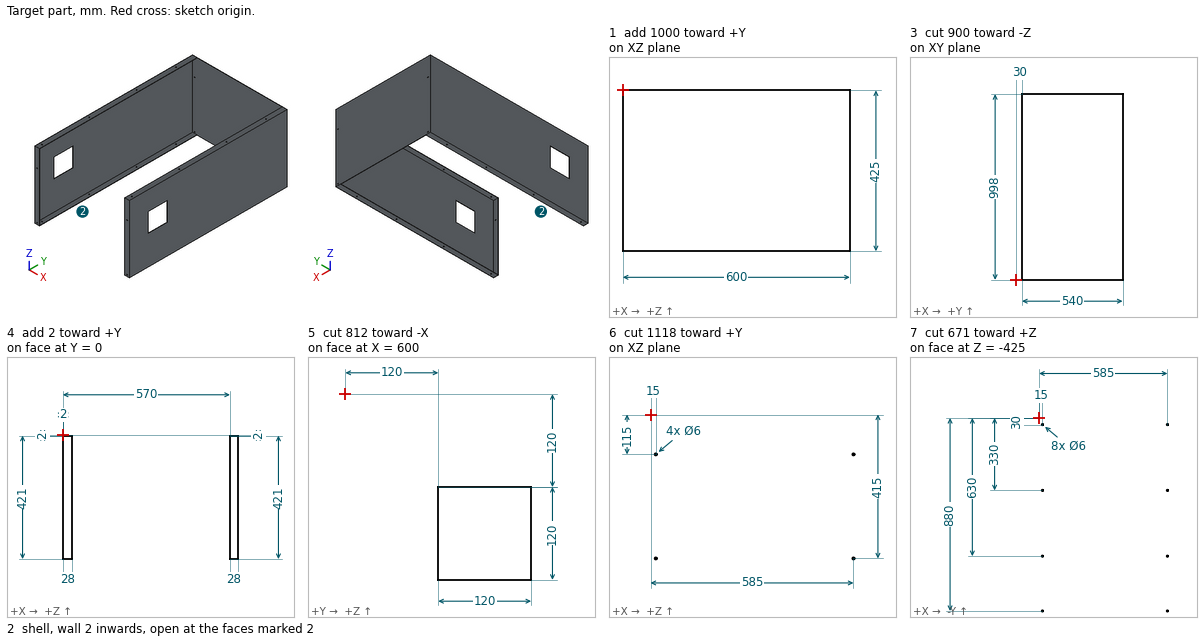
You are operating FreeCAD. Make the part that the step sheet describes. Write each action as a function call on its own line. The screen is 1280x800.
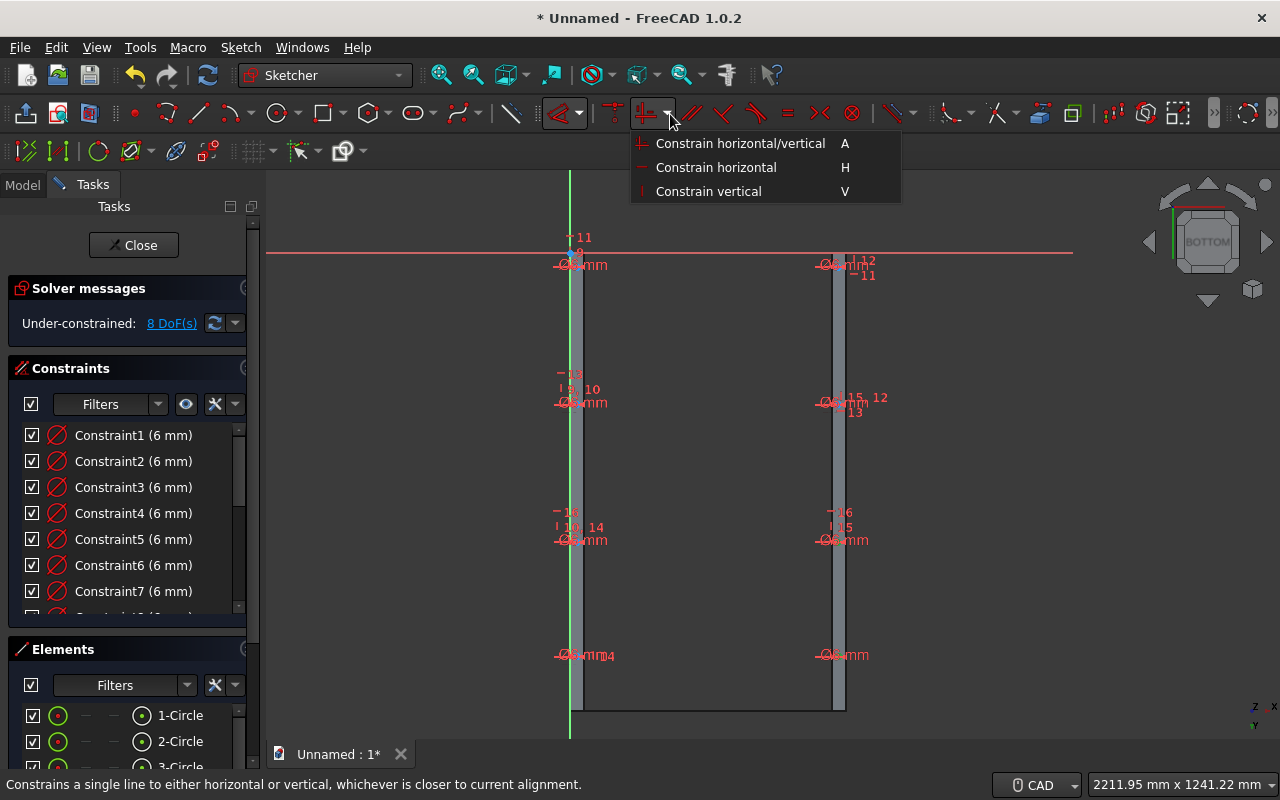
click(766, 191)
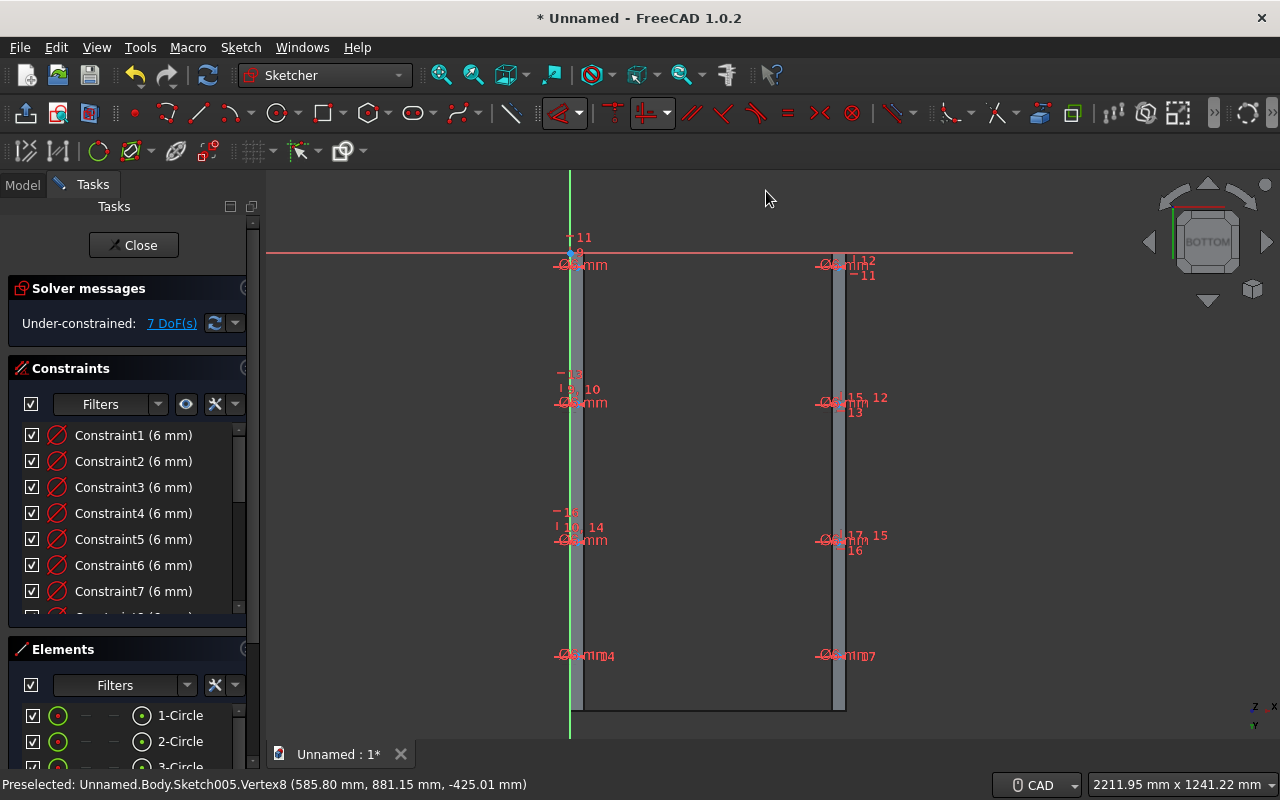
click(577, 657)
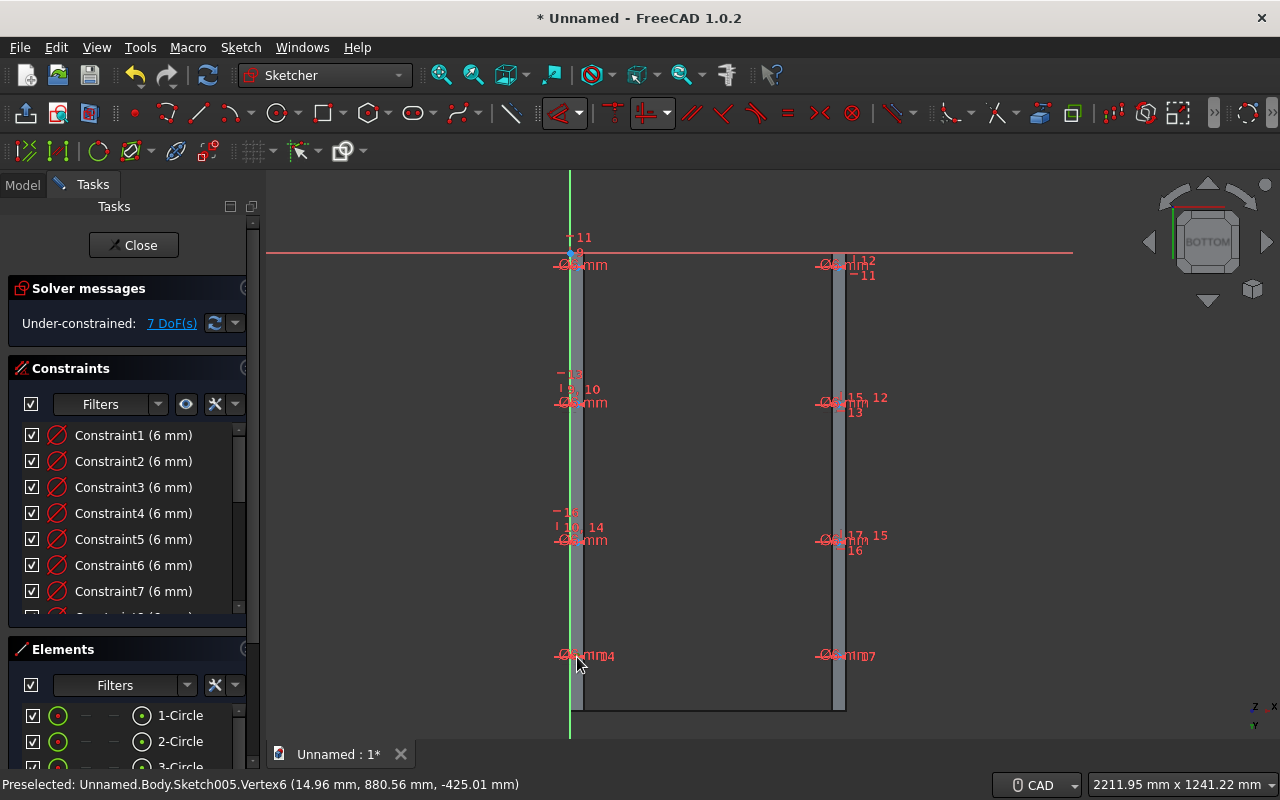
click(838, 657)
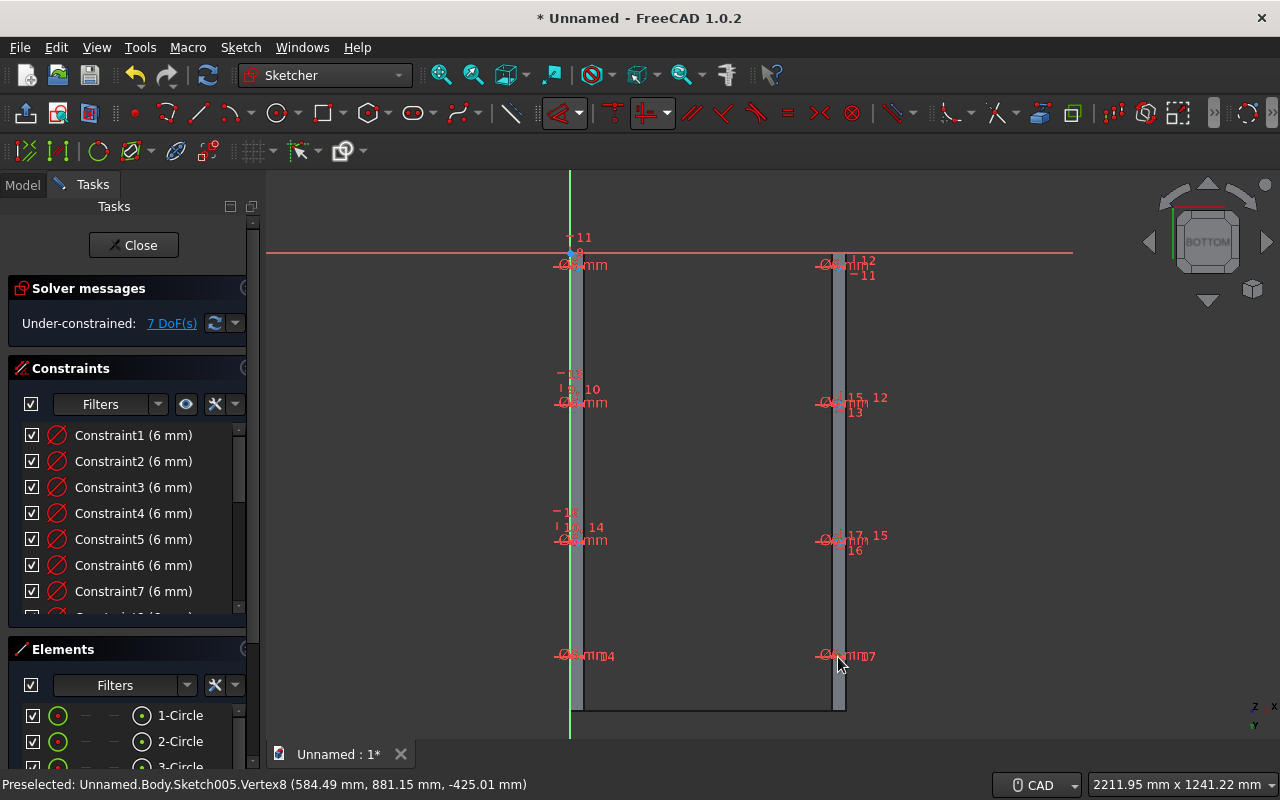
click(670, 114)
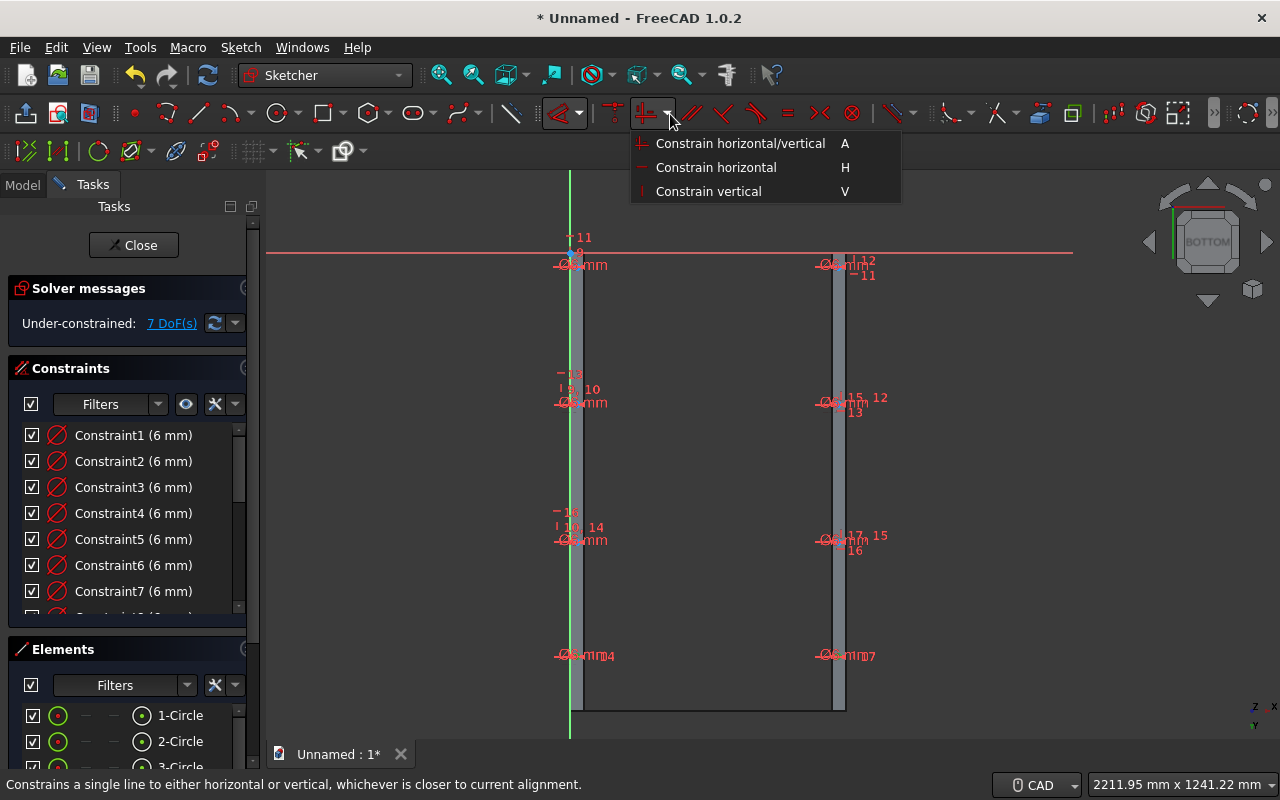
click(766, 167)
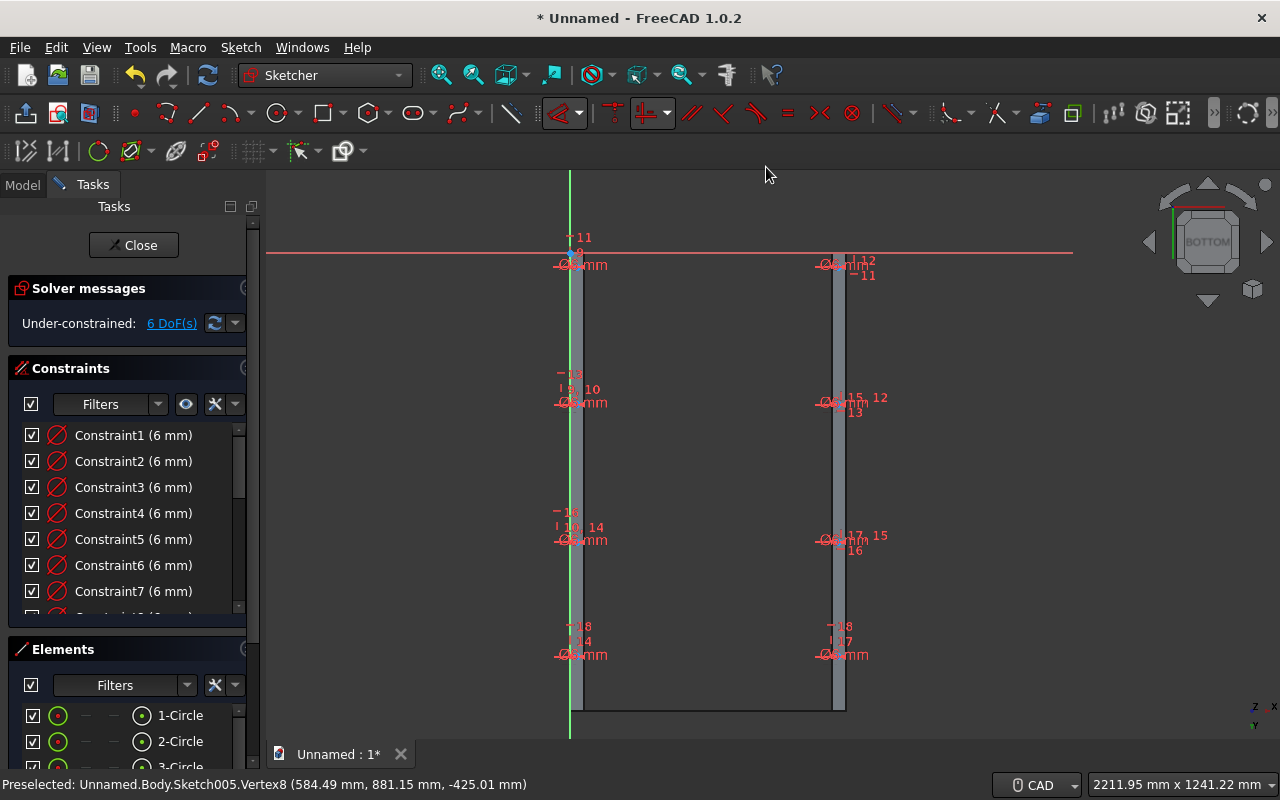
scroll(577, 267, up, 9)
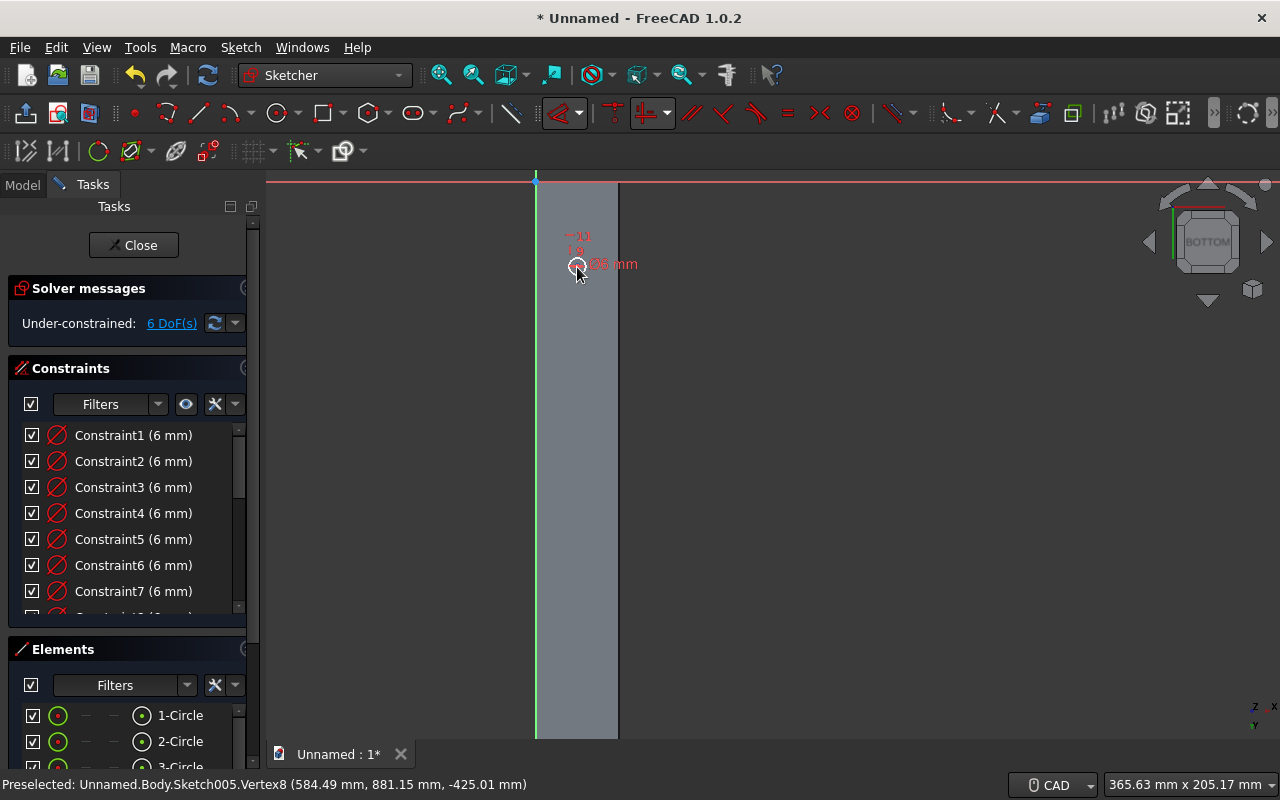
click(577, 266)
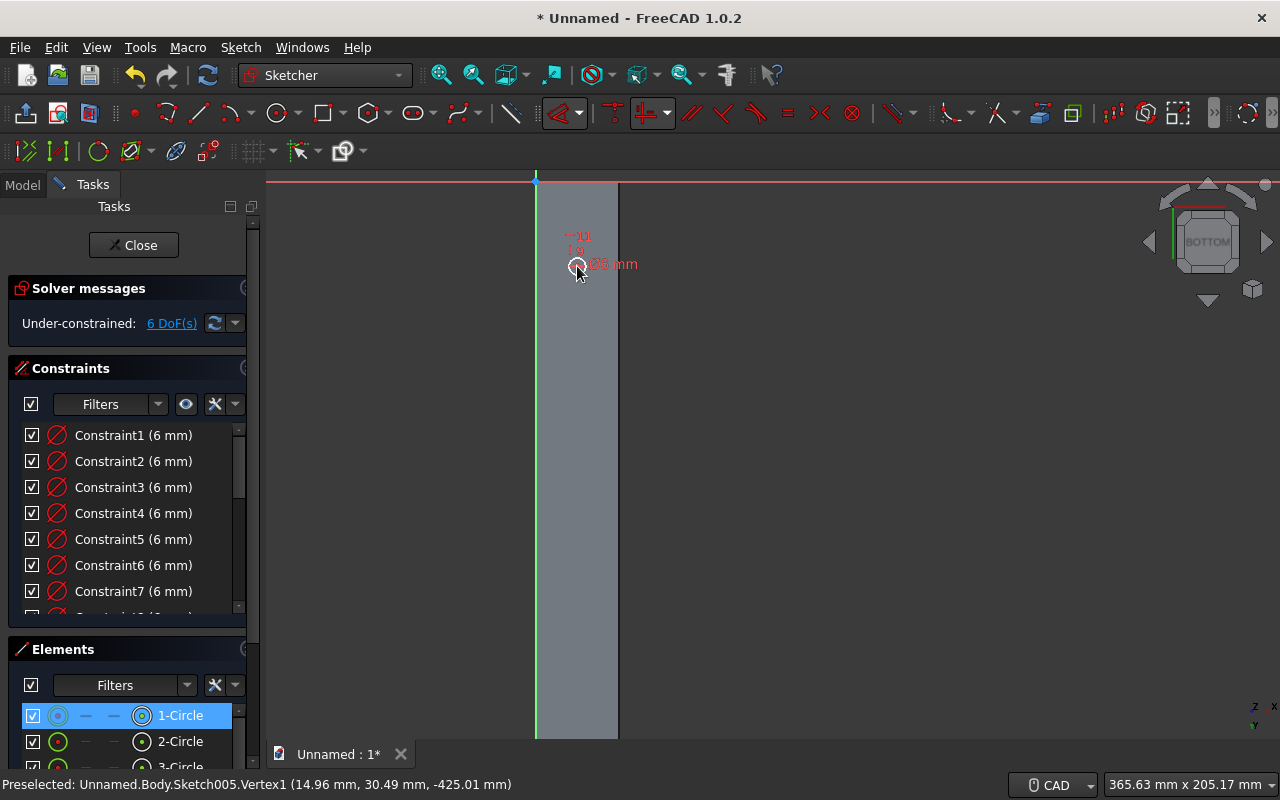
key(l)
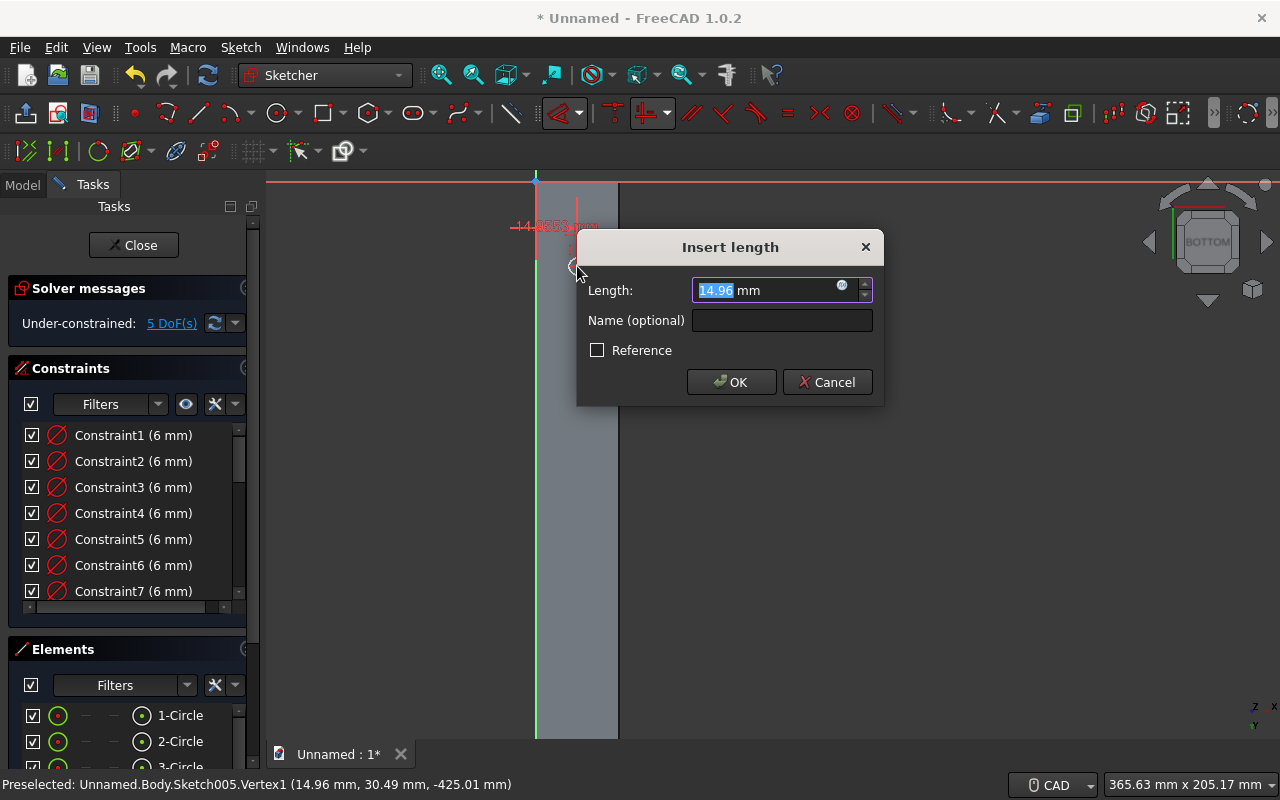
text(15)
key(Return)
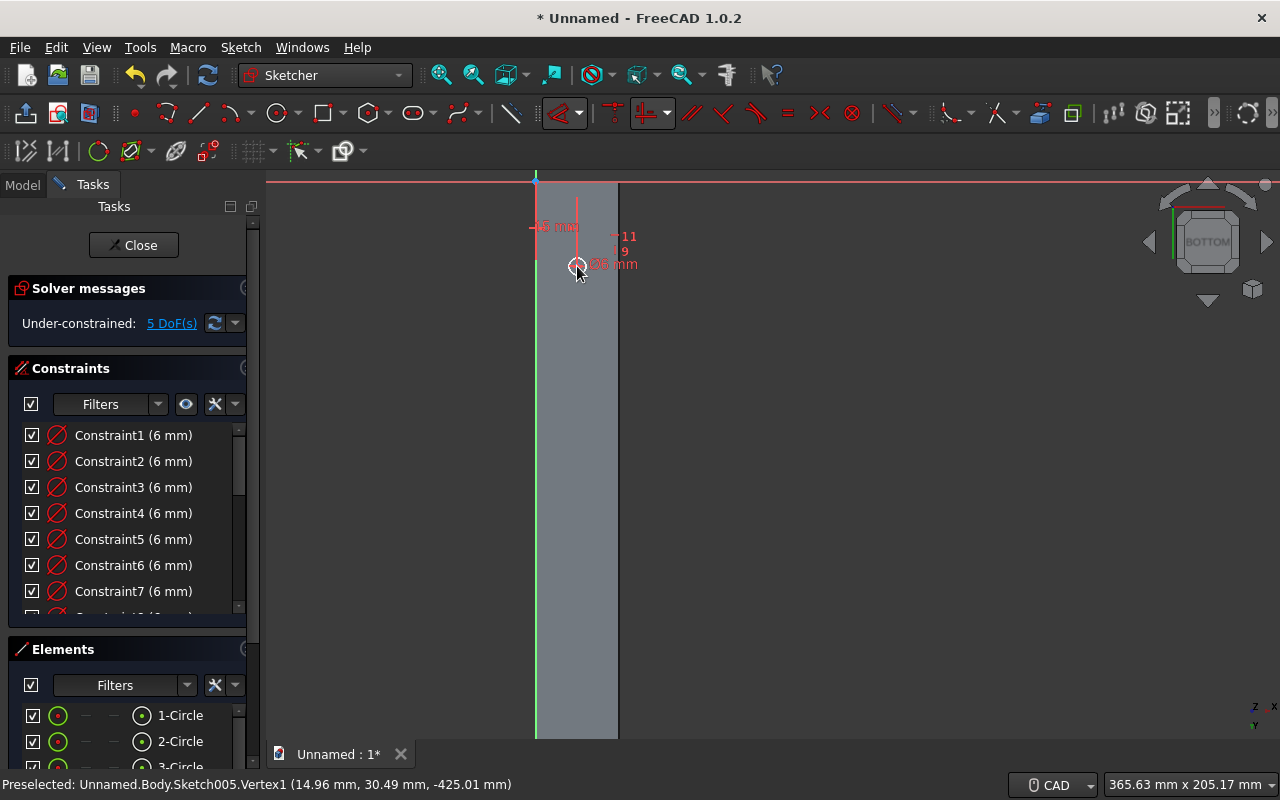
click(577, 266)